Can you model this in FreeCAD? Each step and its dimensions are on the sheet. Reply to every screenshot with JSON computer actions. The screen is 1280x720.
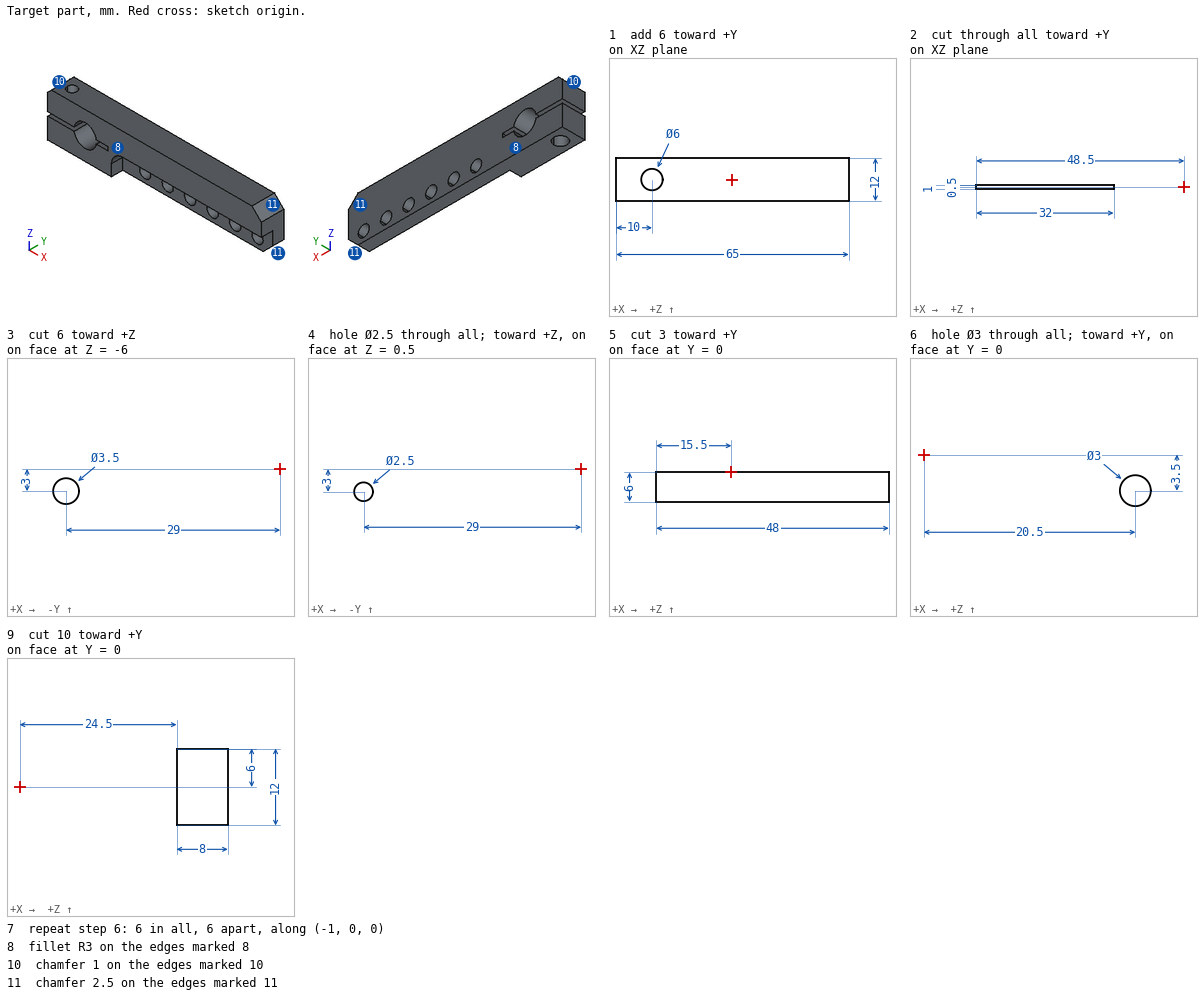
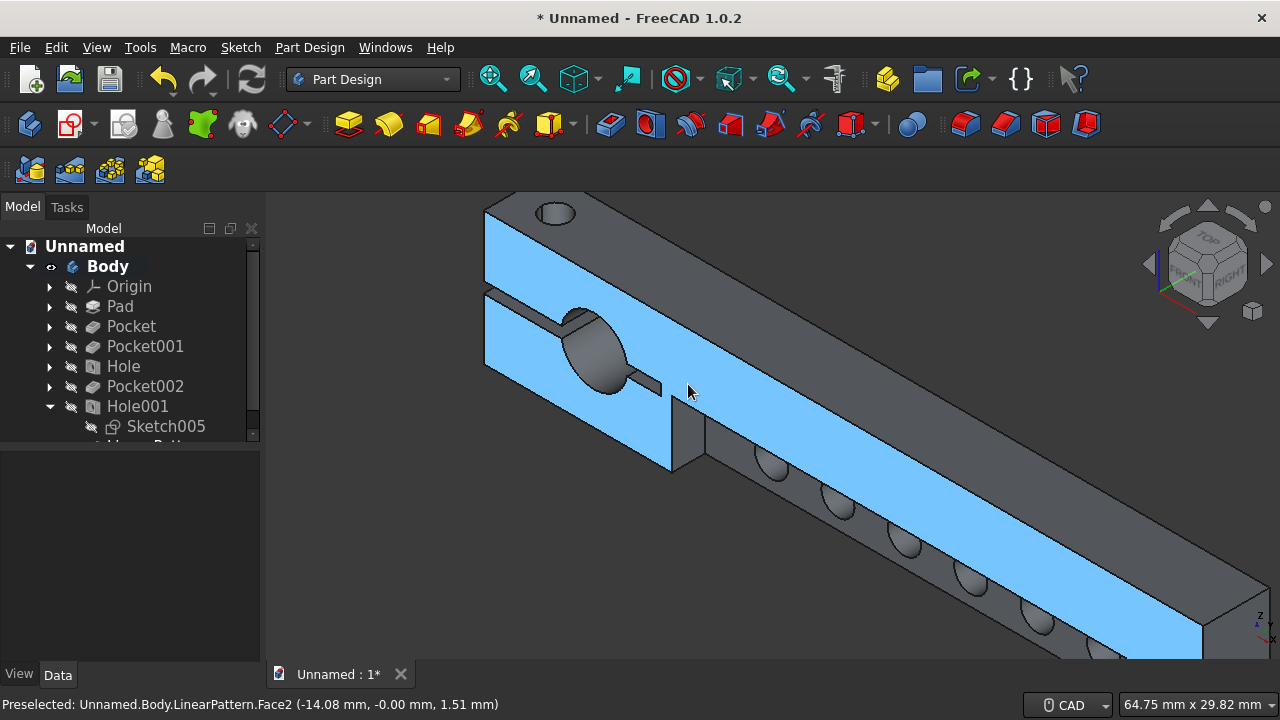
{"action": "left_click", "coordinate": [494, 80]}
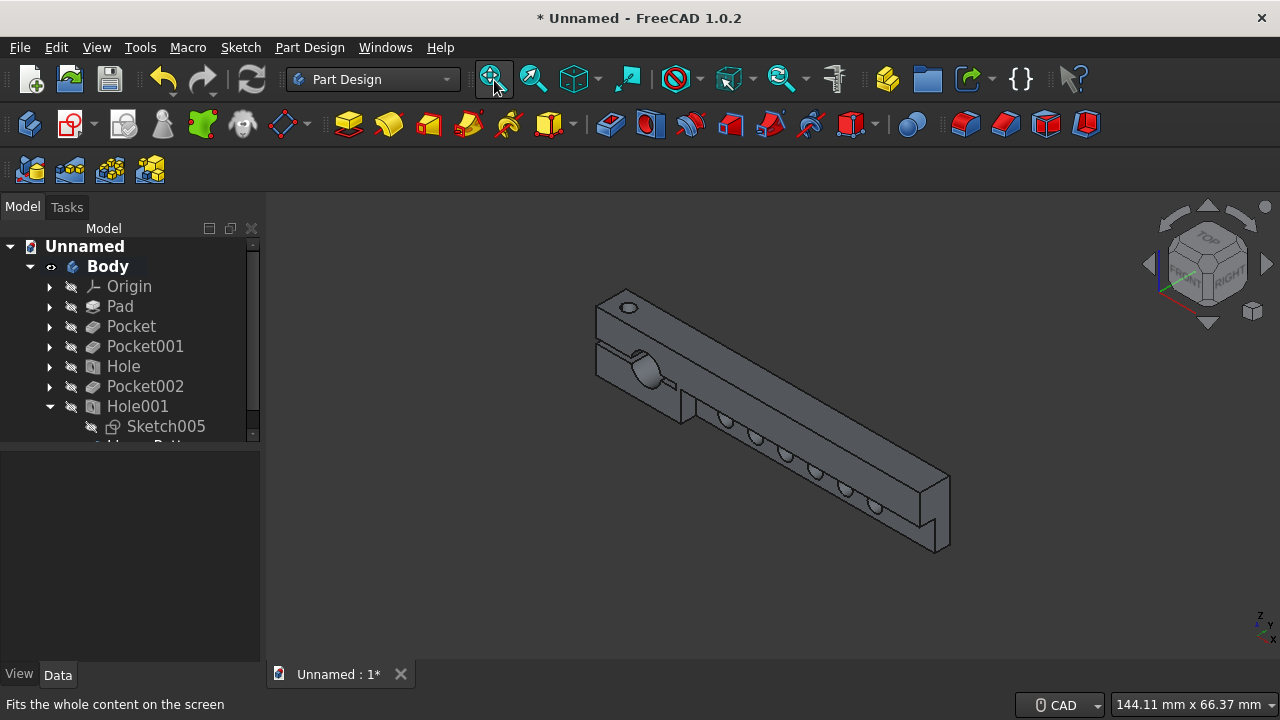
{"action": "key", "text": "2"}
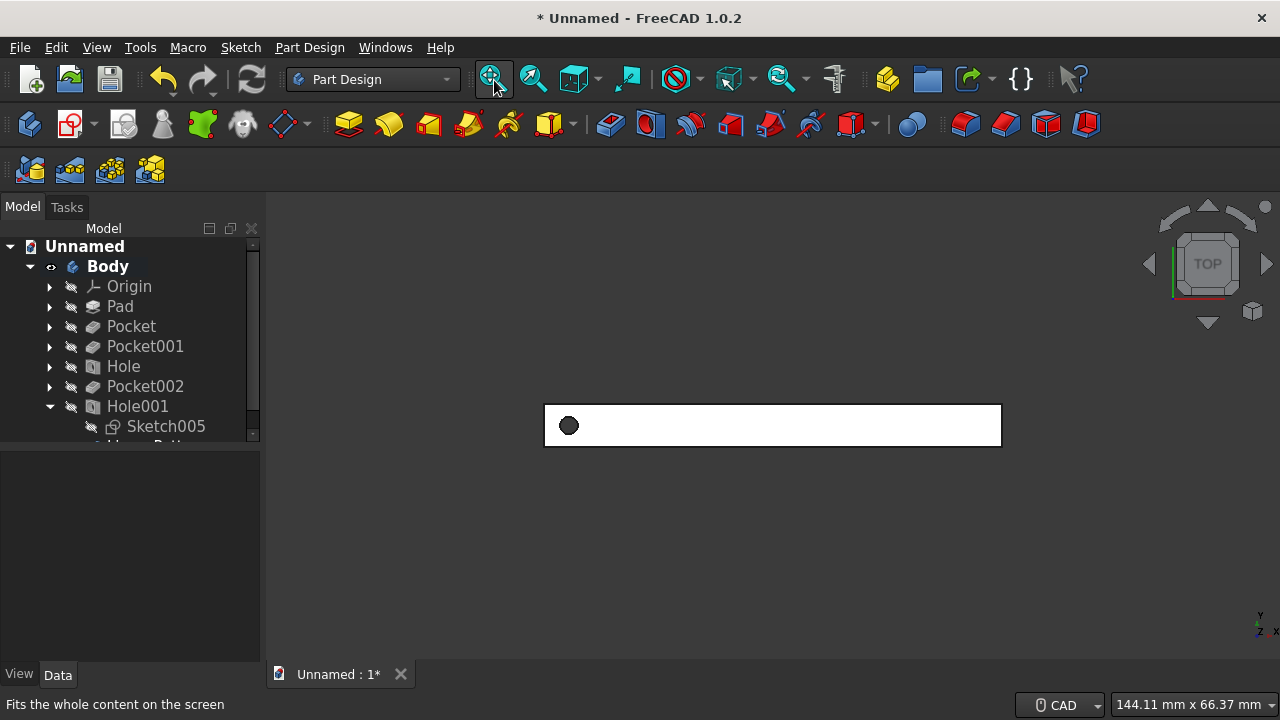
{"action": "scroll", "coordinate": [664, 435], "scroll_direction": "up", "scroll_amount": 4}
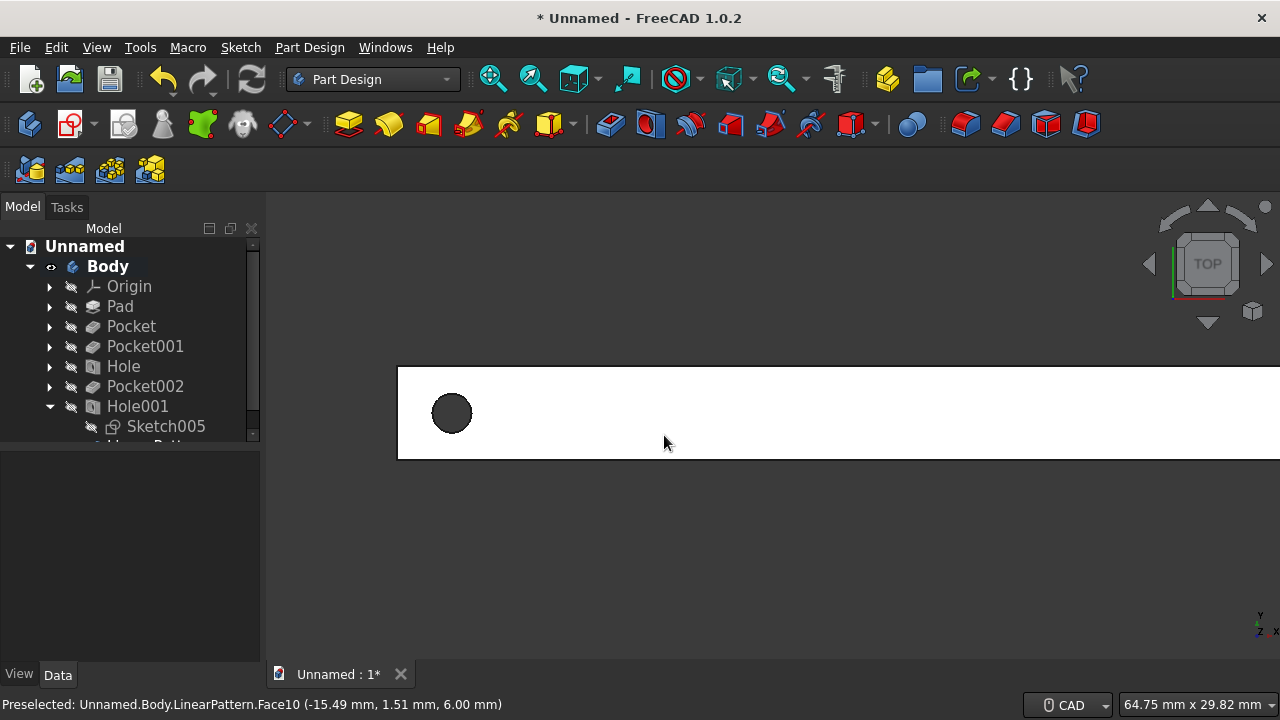
{"action": "left_click", "coordinate": [494, 80]}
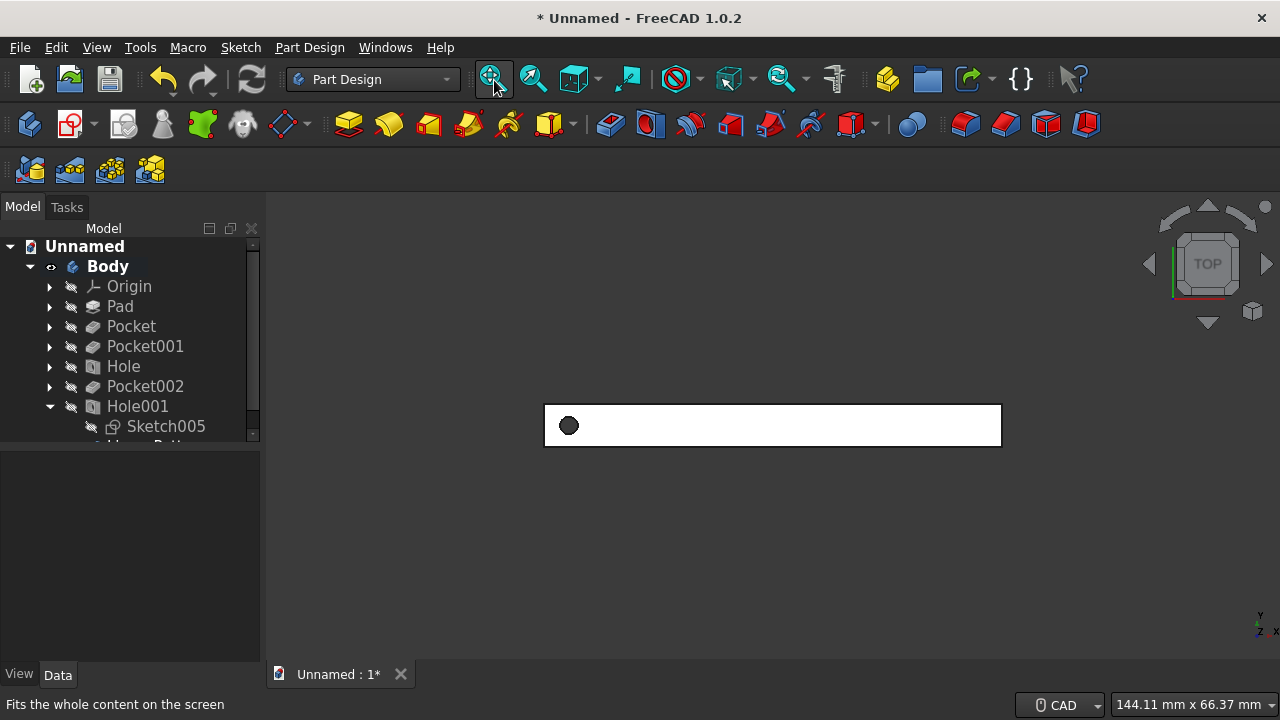
{"action": "key", "text": "0"}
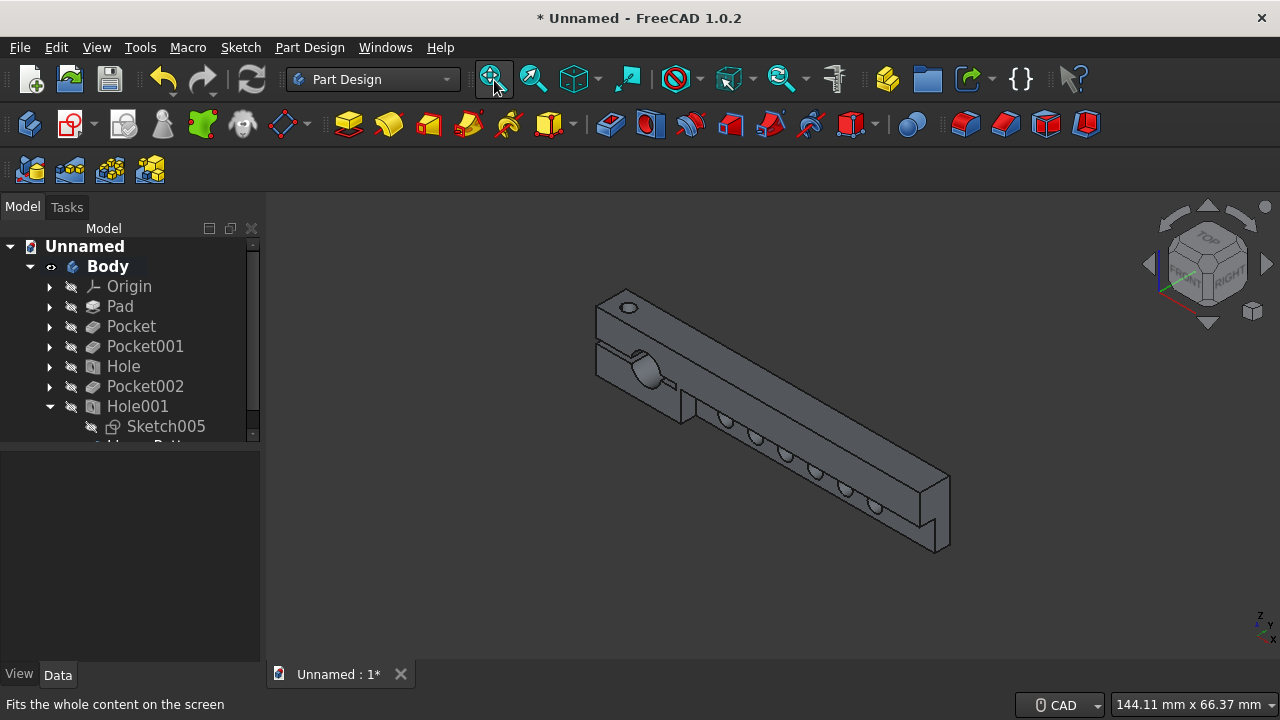
{"action": "scroll", "coordinate": [688, 384], "scroll_direction": "up", "scroll_amount": 4}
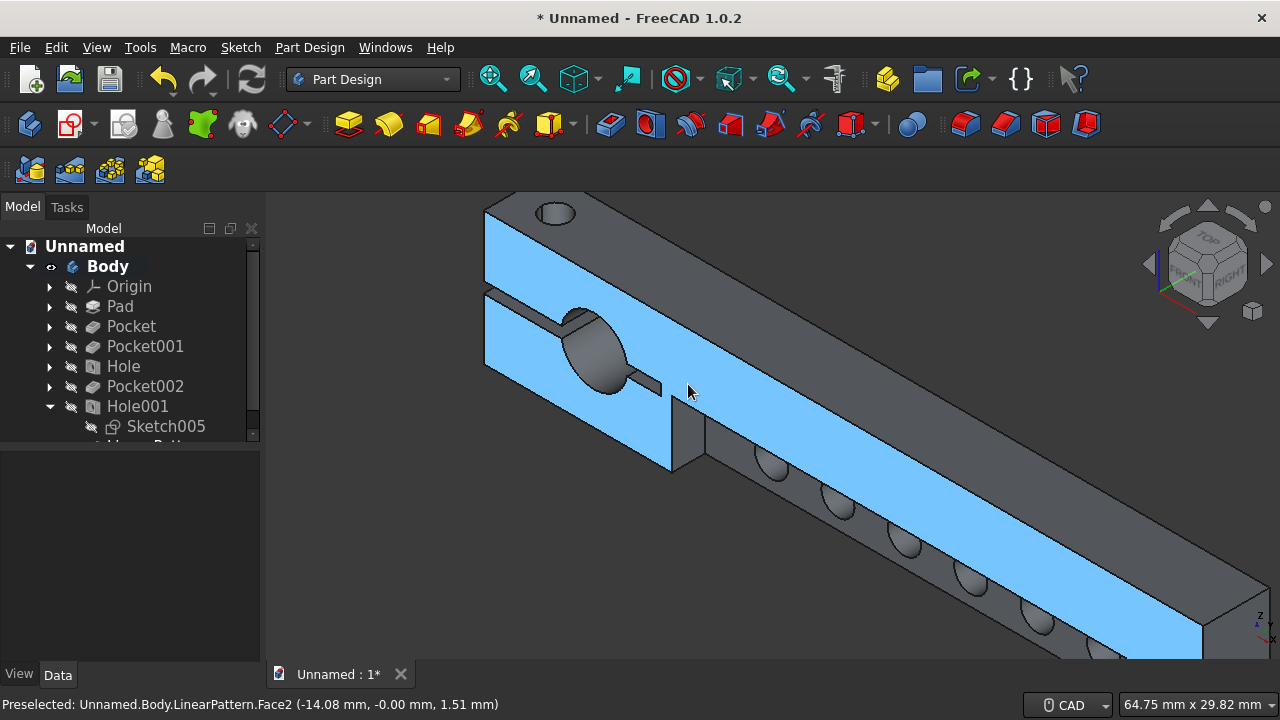
{"action": "key", "text": "v f"}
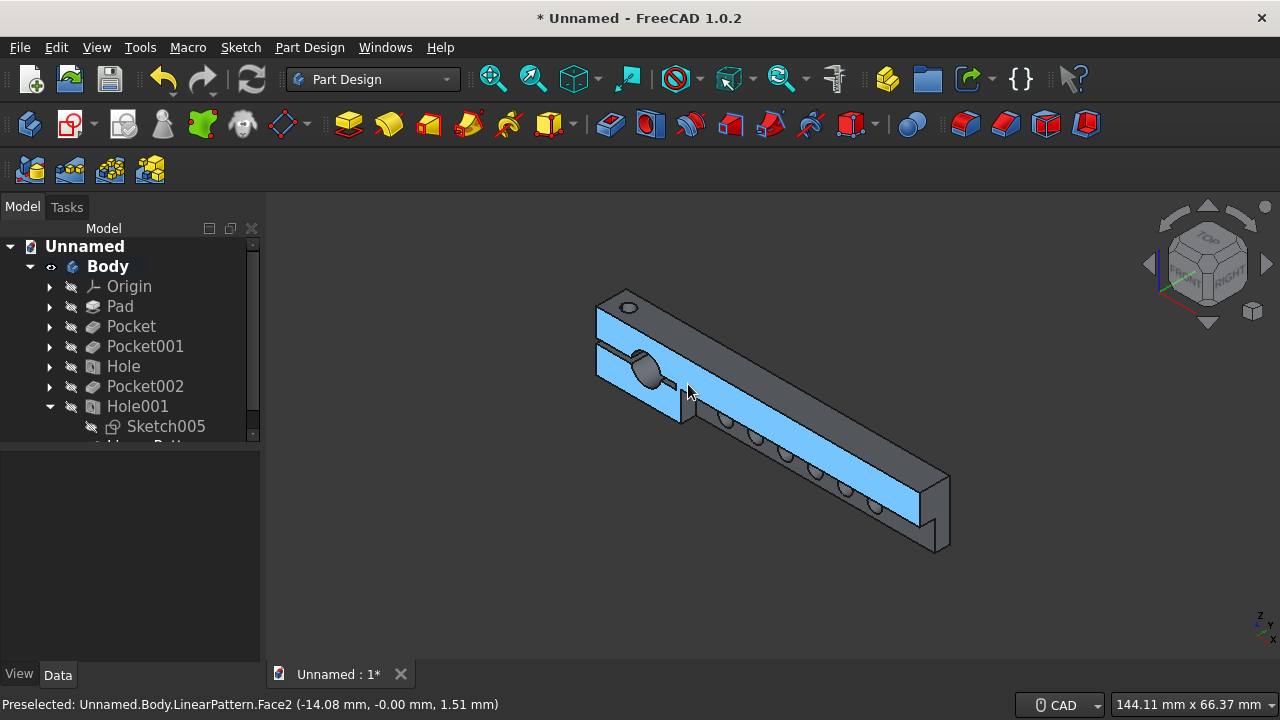
{"action": "key", "text": "1"}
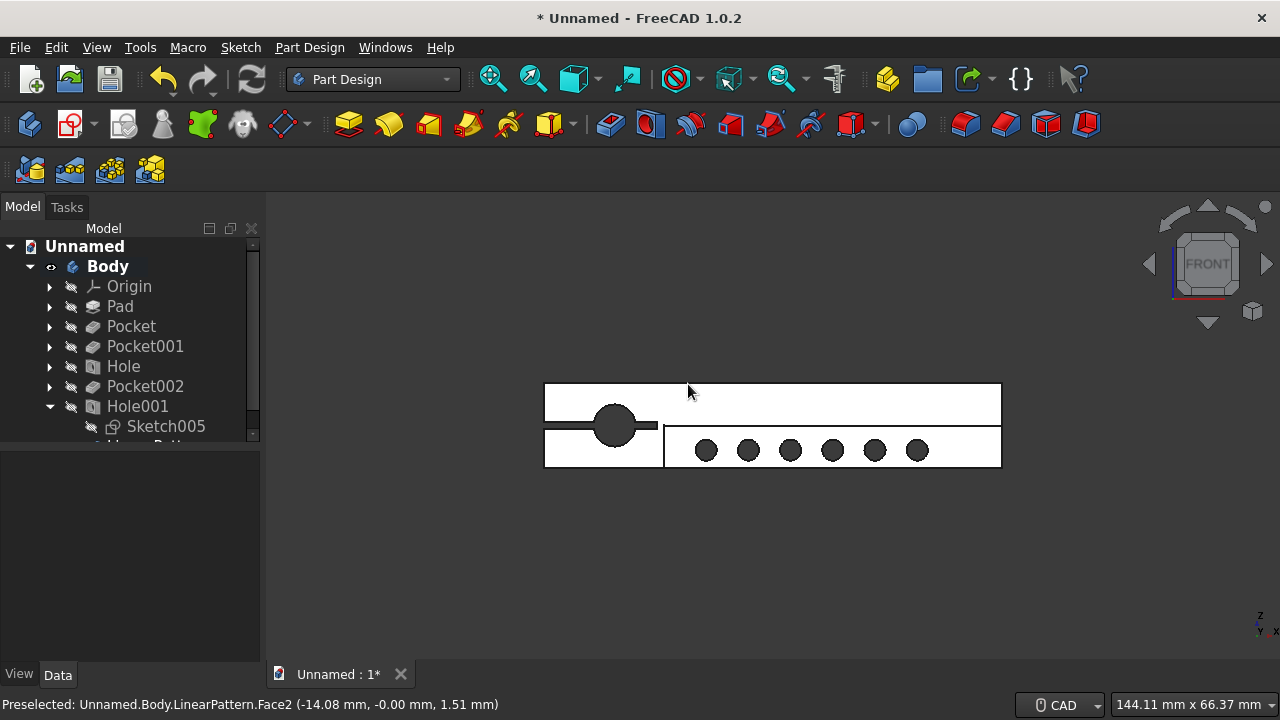
{"action": "scroll", "coordinate": [664, 424], "scroll_direction": "up", "scroll_amount": 4}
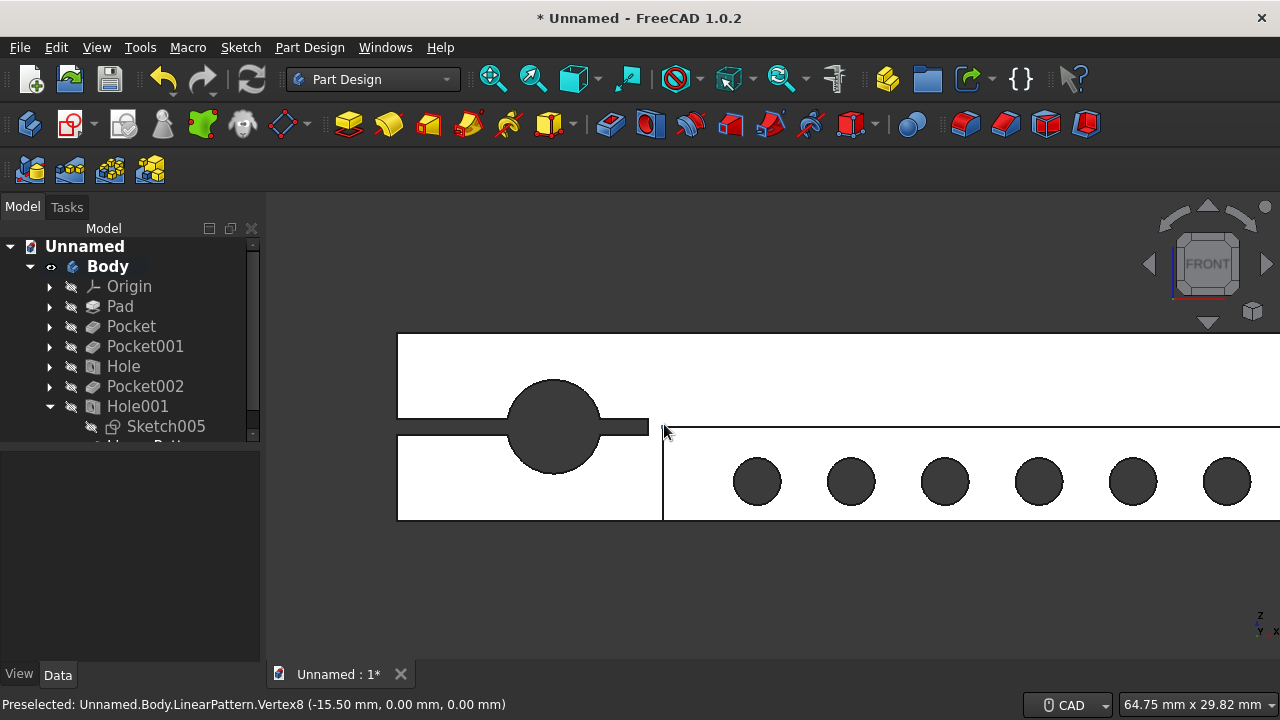
{"action": "left_click", "coordinate": [494, 80]}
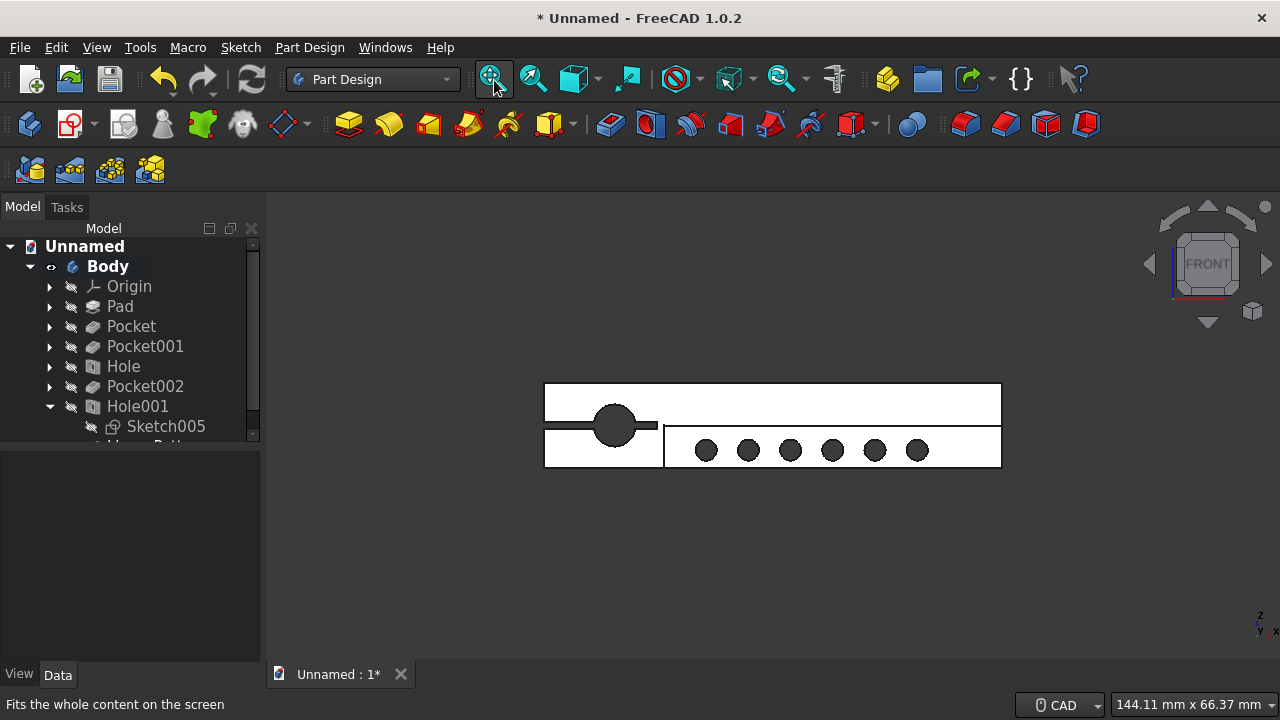
{"action": "key", "text": "3"}